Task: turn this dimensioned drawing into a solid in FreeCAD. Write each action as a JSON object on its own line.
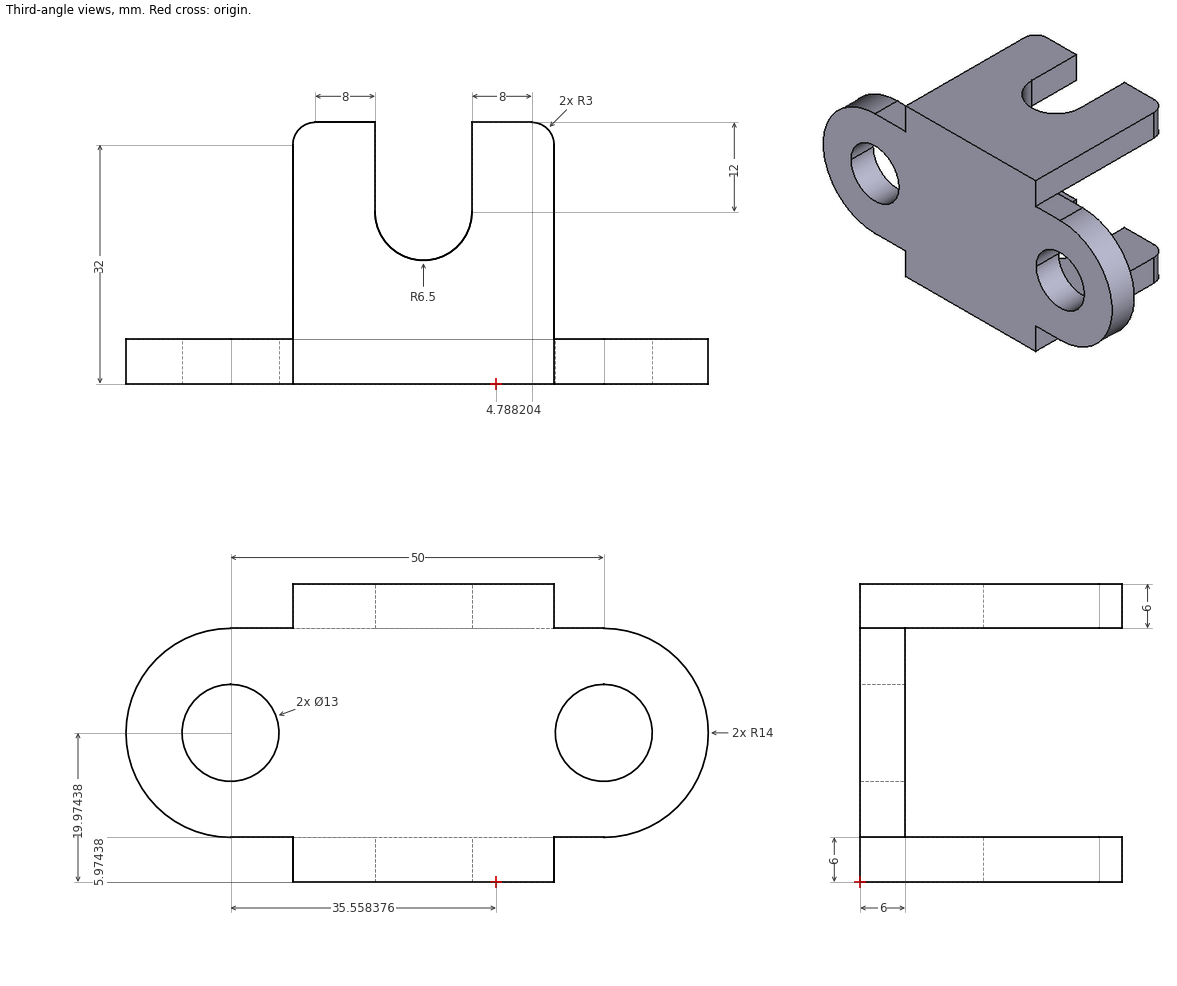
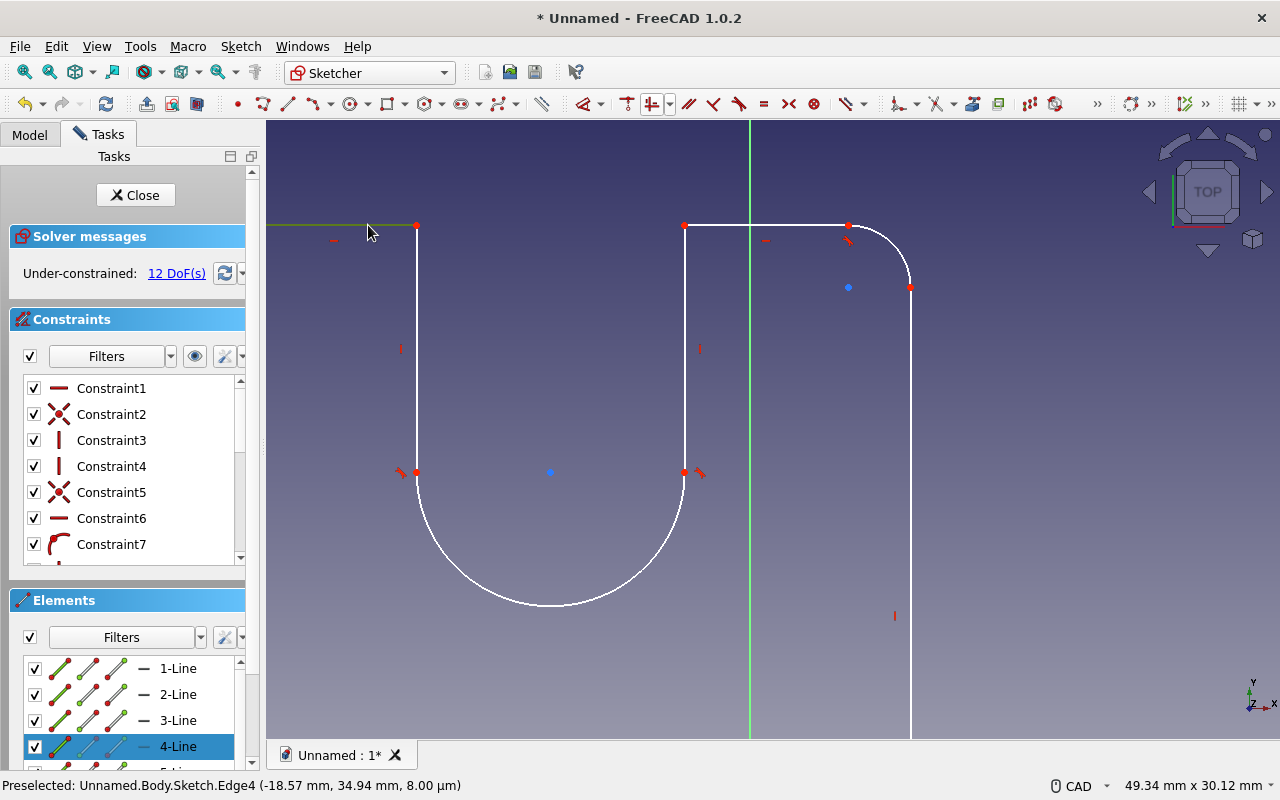
{"action": "scroll", "coordinate": [892, 242], "scroll_direction": "down", "scroll_amount": 3}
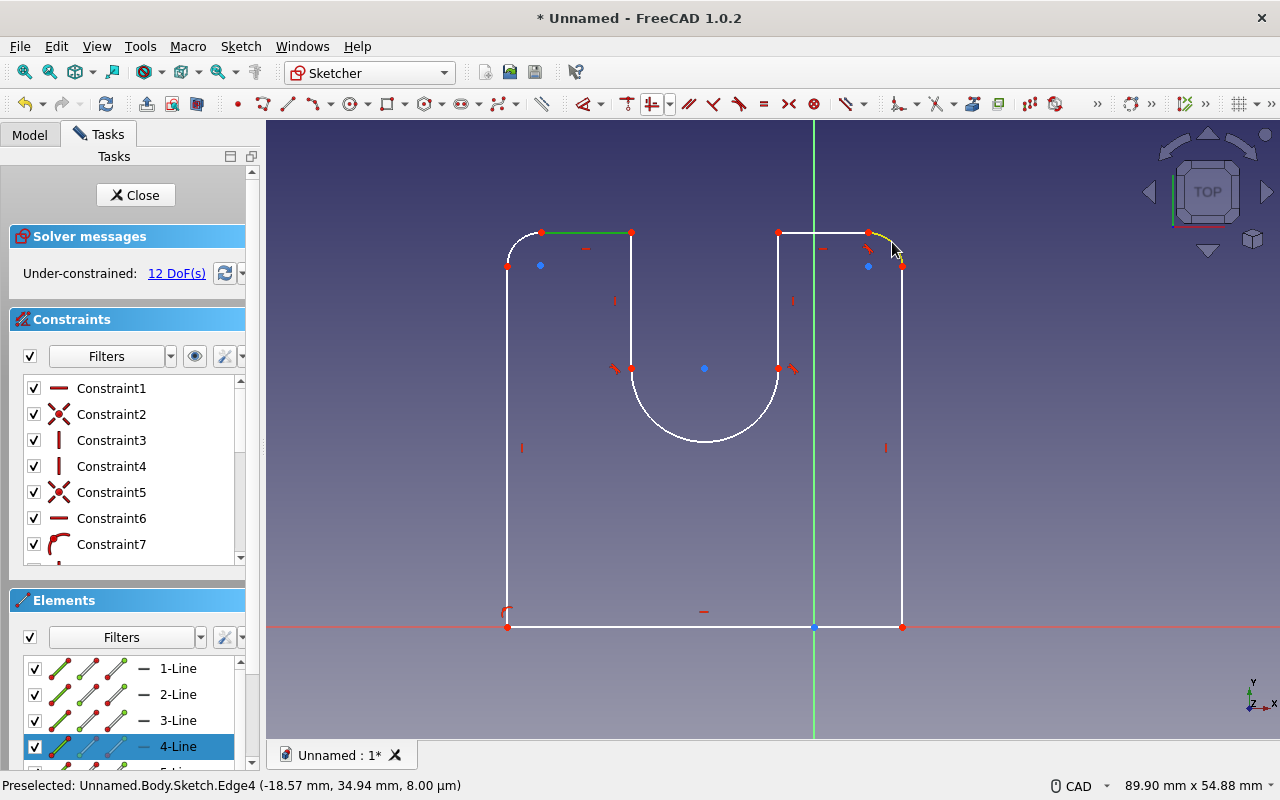
{"action": "left_click", "coordinate": [526, 236]}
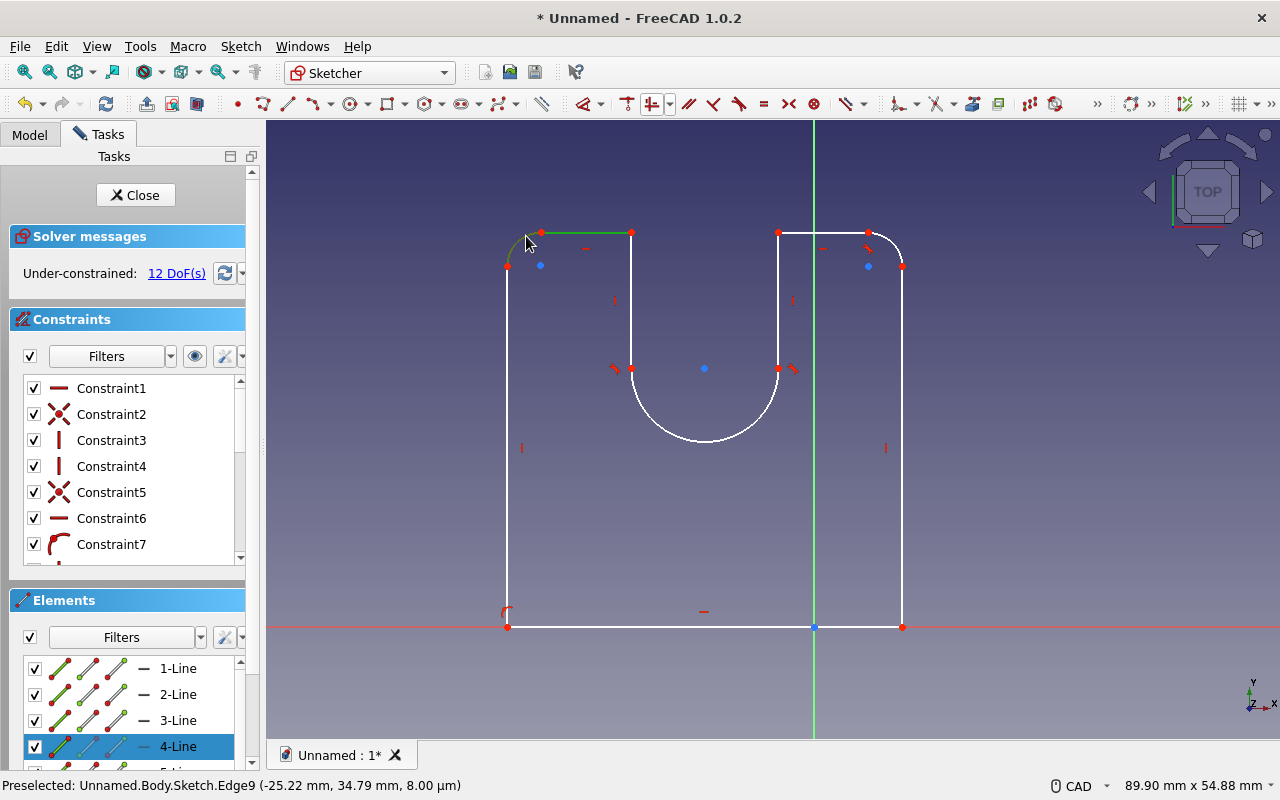
{"action": "left_click", "coordinate": [739, 104]}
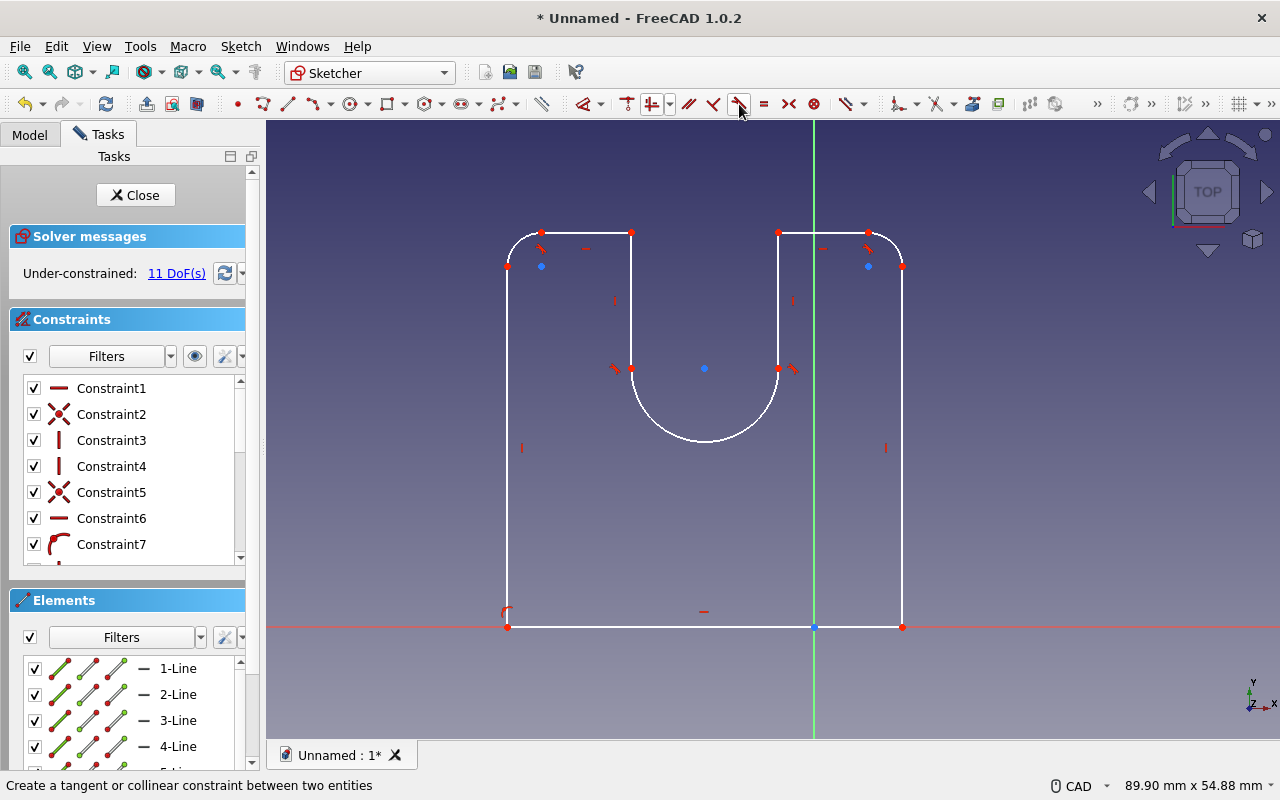
{"action": "left_click", "coordinate": [507, 375]}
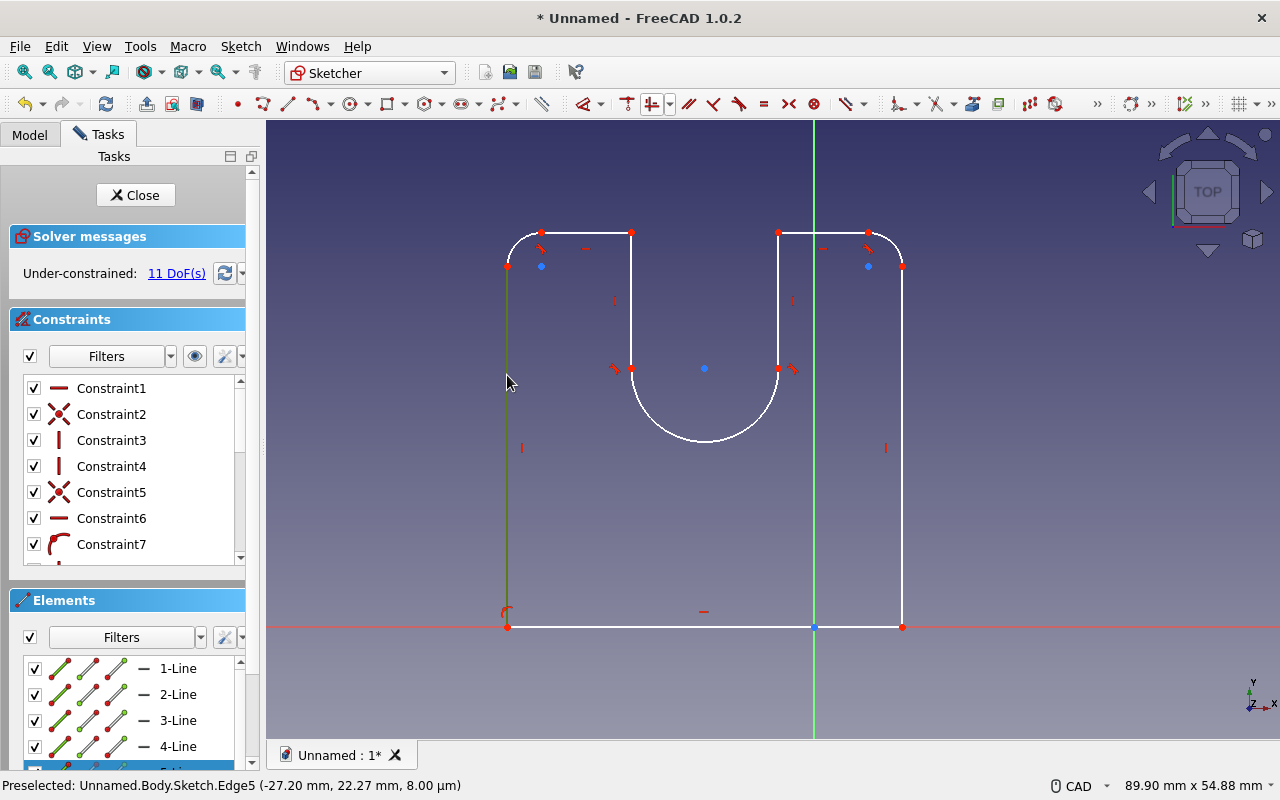
{"action": "left_click", "coordinate": [526, 237]}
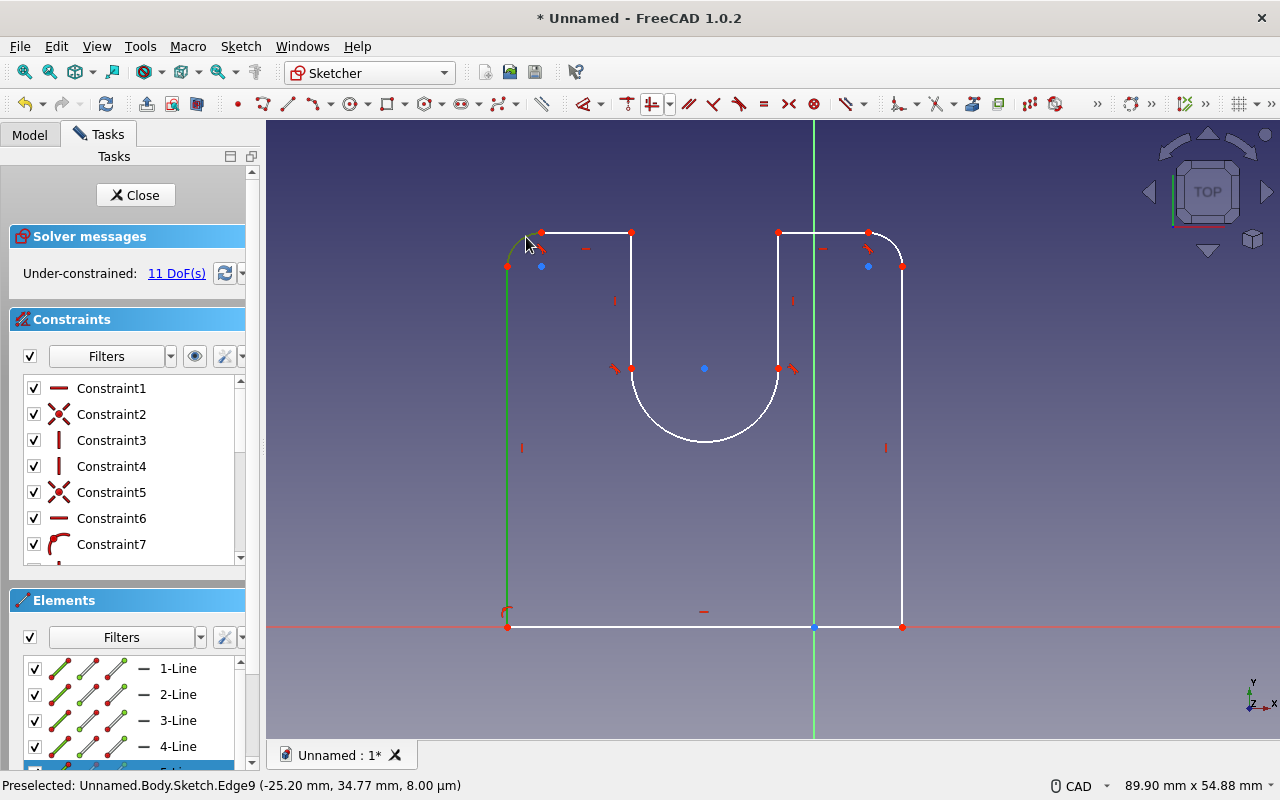
{"action": "left_click", "coordinate": [739, 104]}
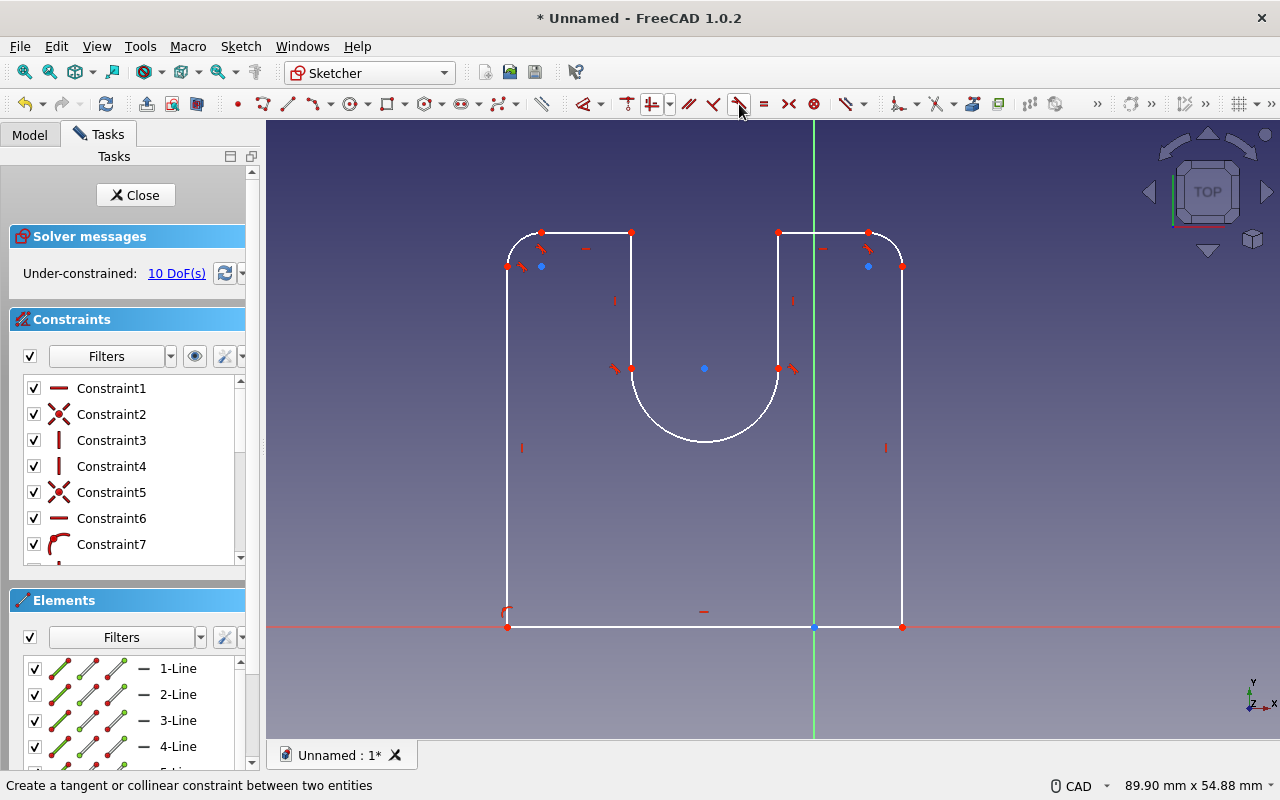
{"action": "left_click", "coordinate": [902, 519]}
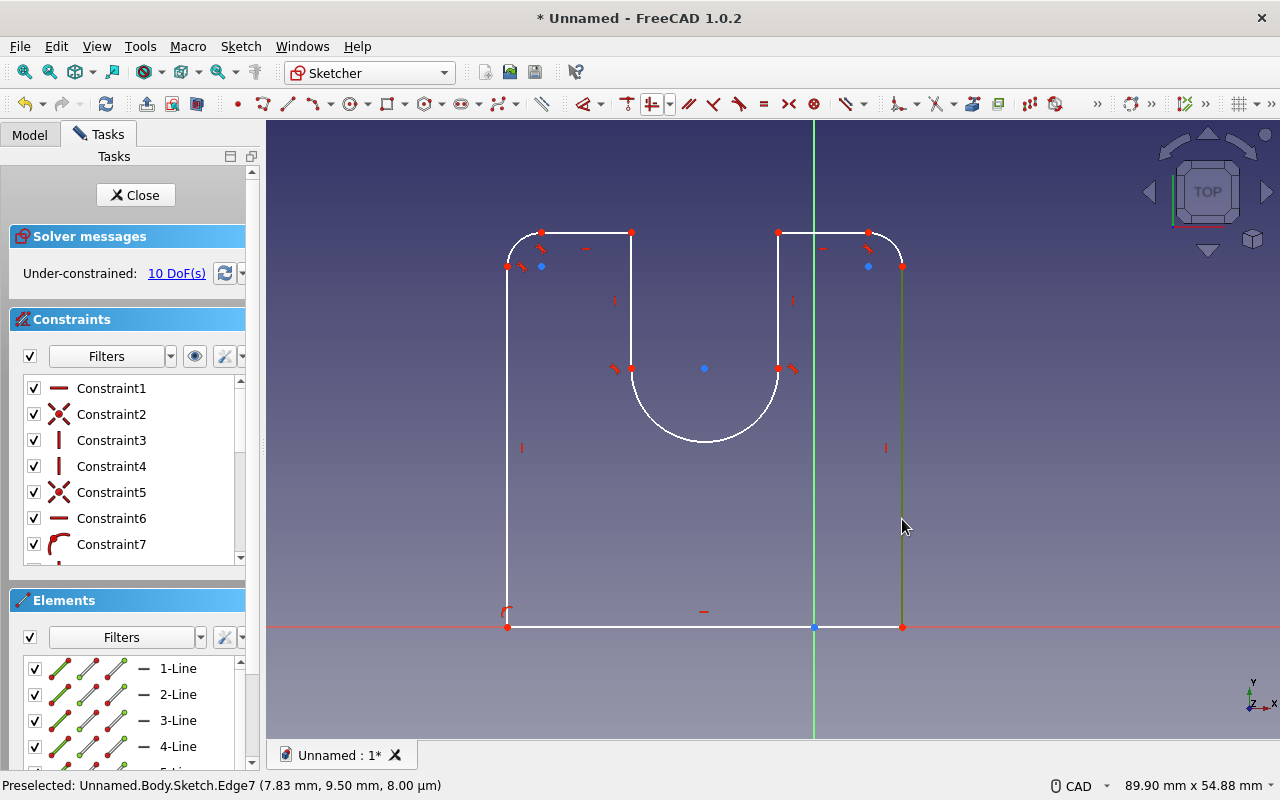
{"action": "left_click", "coordinate": [899, 252]}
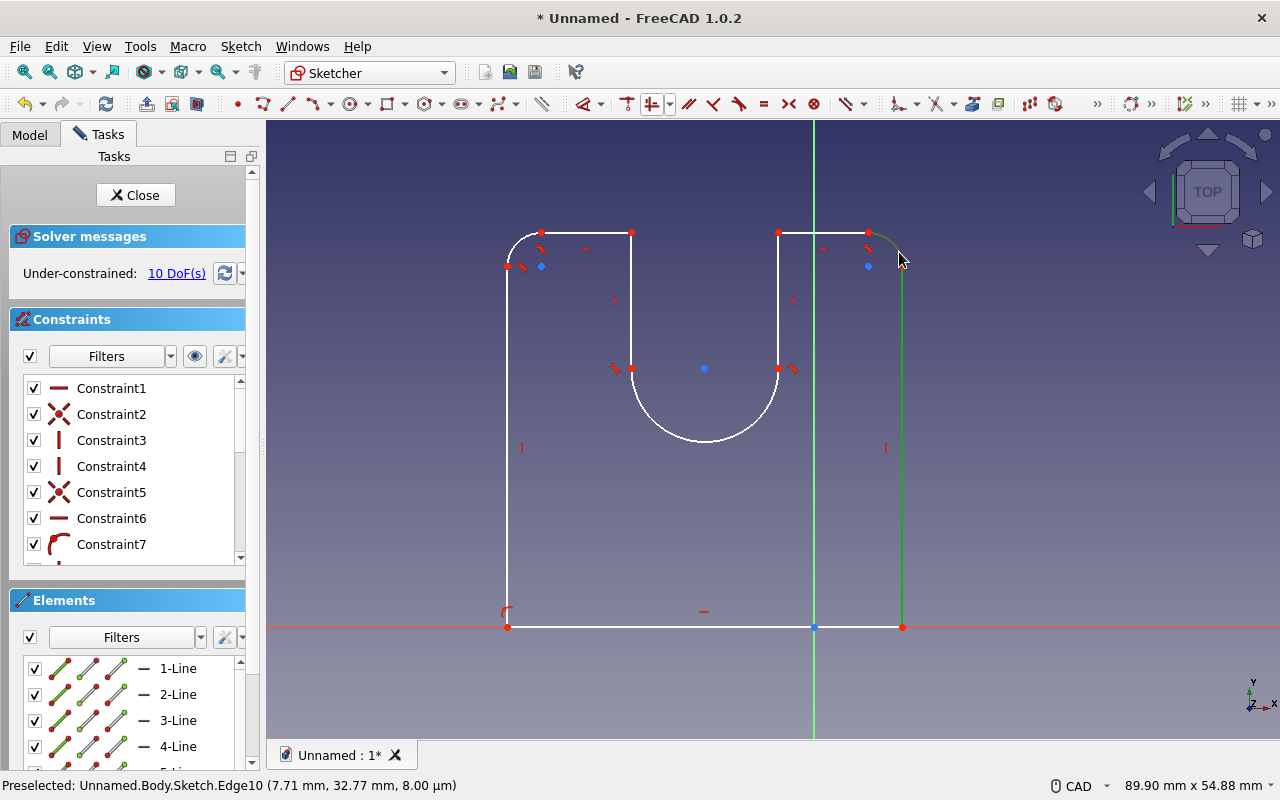
{"action": "left_click", "coordinate": [739, 104]}